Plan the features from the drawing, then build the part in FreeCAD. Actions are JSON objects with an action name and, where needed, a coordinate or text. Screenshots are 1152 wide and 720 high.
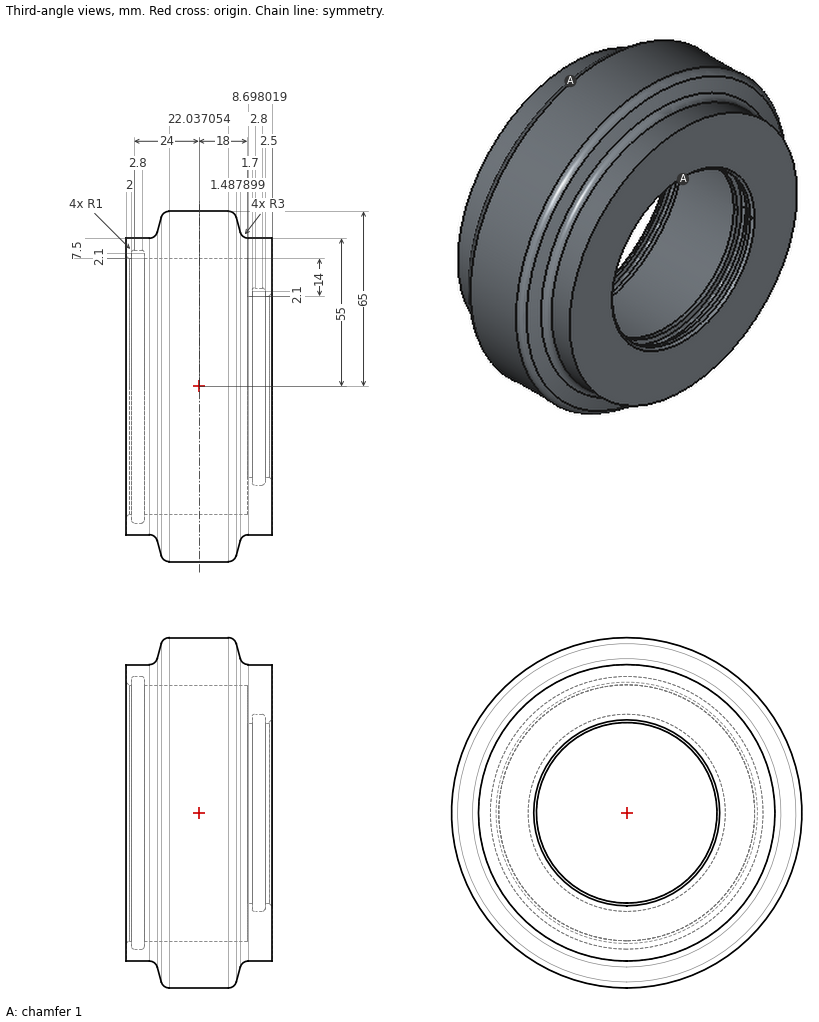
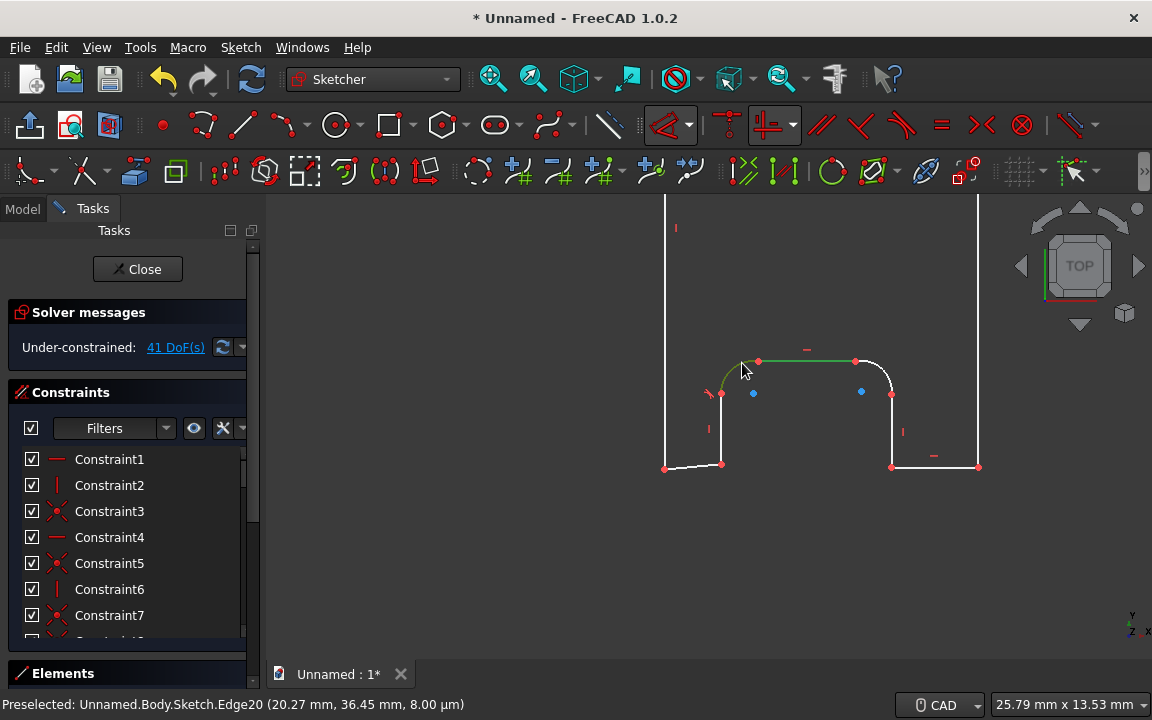
{"action": "key", "text": "t"}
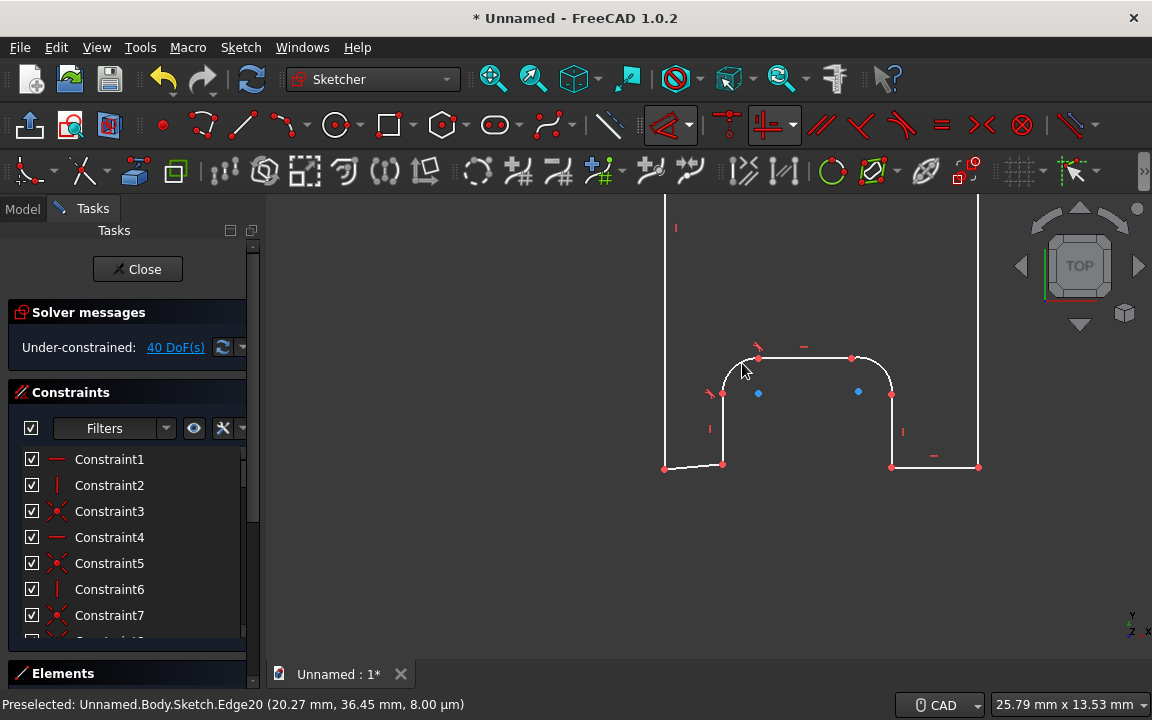
{"action": "left_click", "coordinate": [786, 358]}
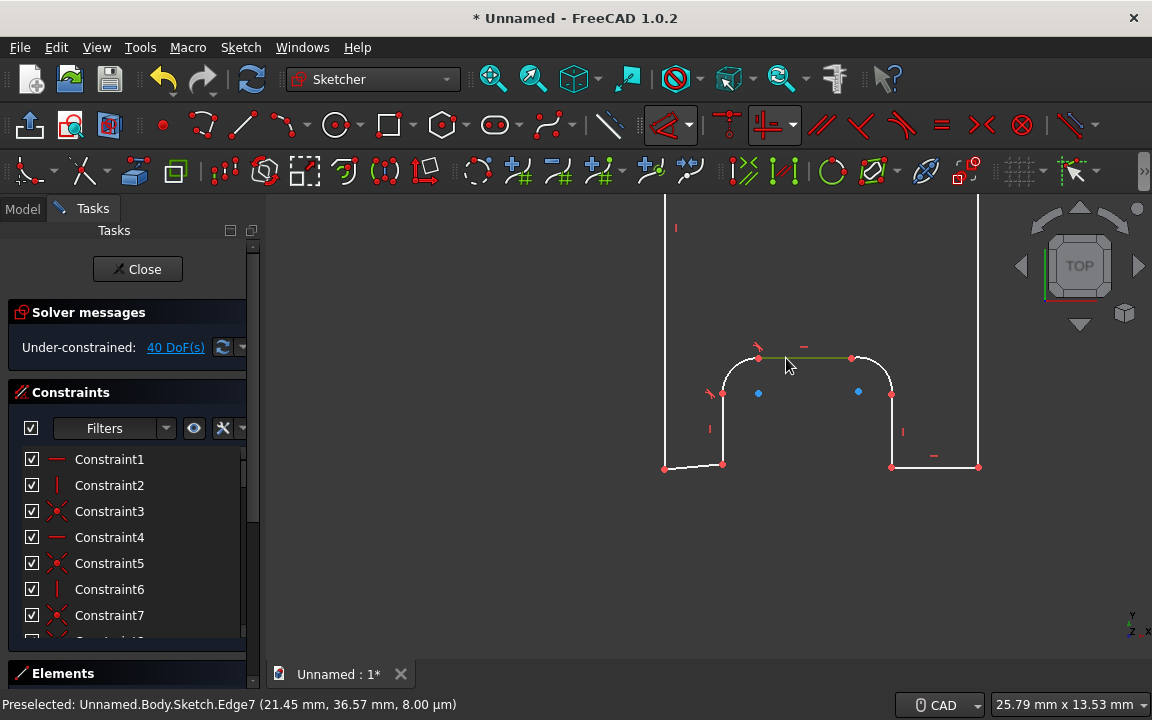
{"action": "left_click", "coordinate": [888, 376]}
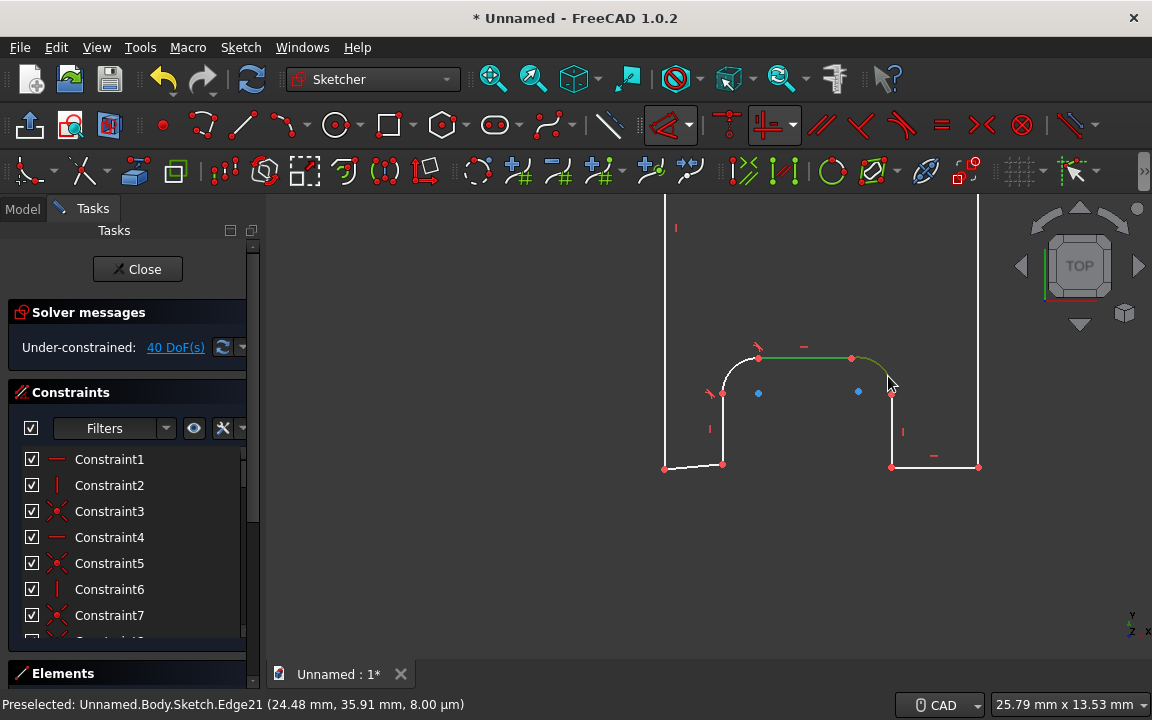
{"action": "key", "text": "t"}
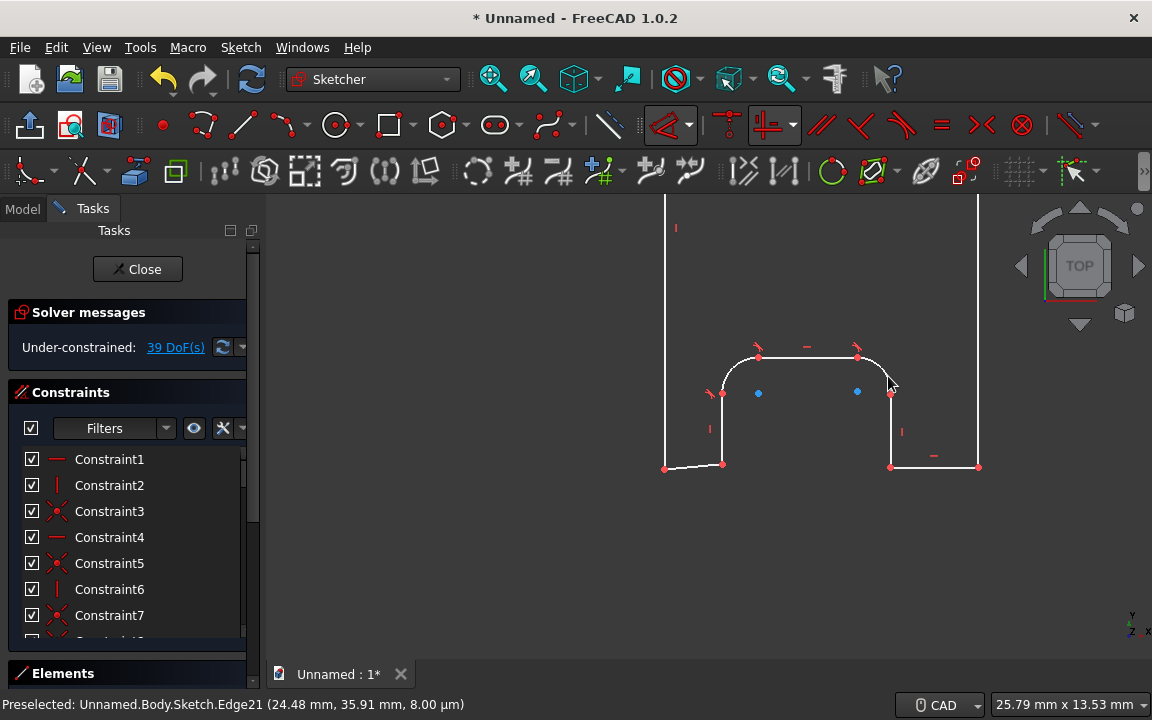
{"action": "left_click", "coordinate": [891, 417]}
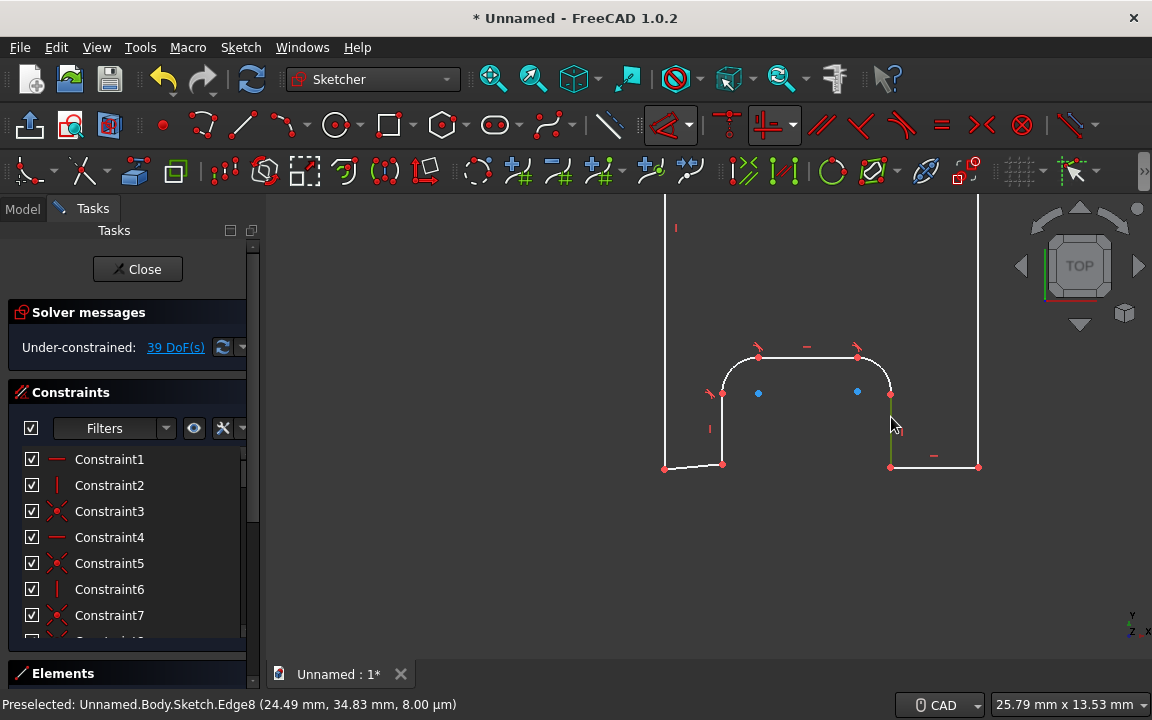
{"action": "left_click", "coordinate": [888, 378]}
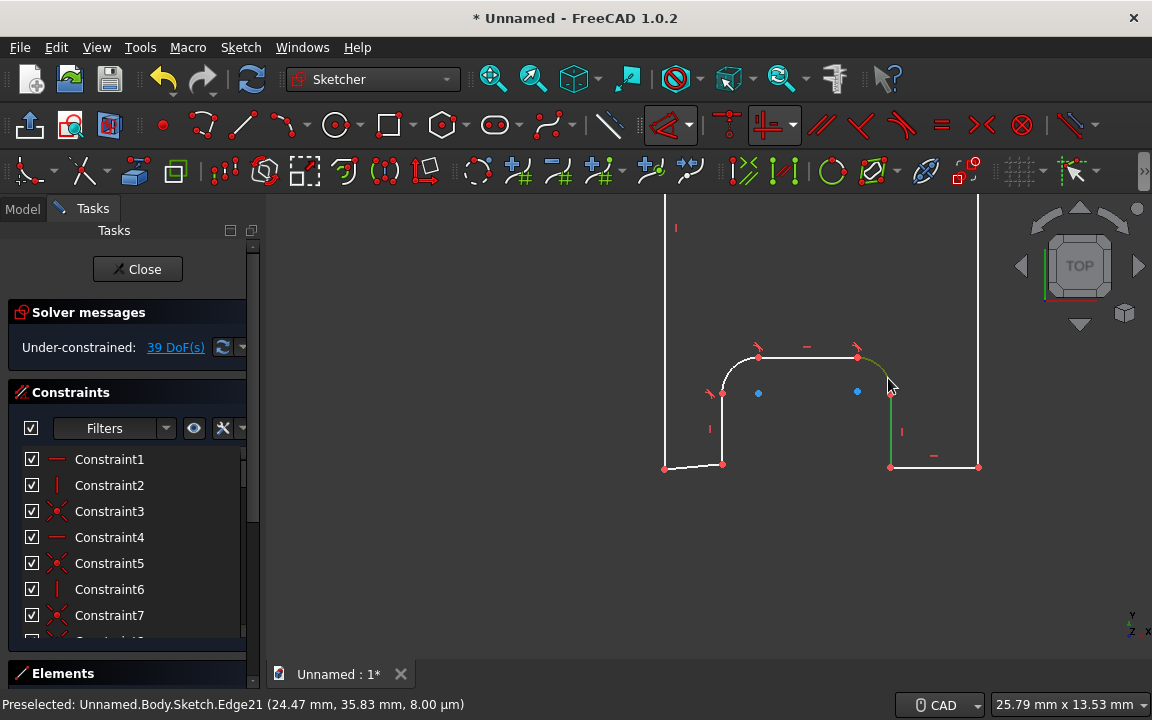
{"action": "key", "text": "t"}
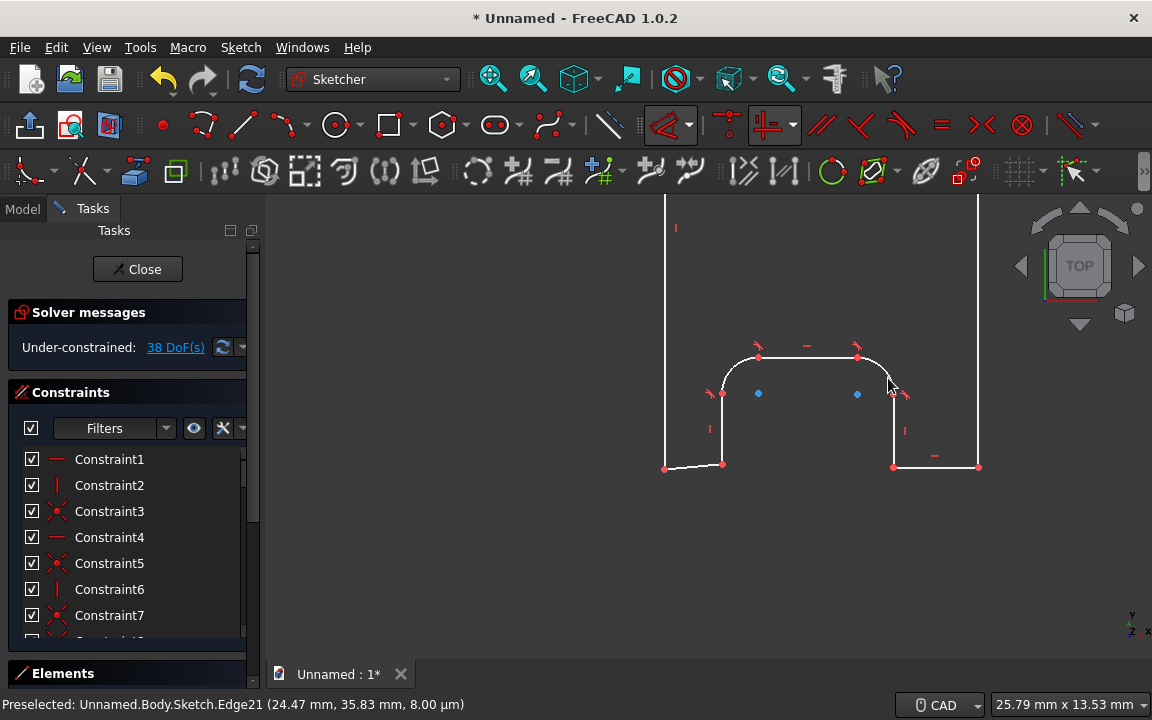
{"action": "scroll", "coordinate": [733, 415], "scroll_direction": "down", "scroll_amount": 10}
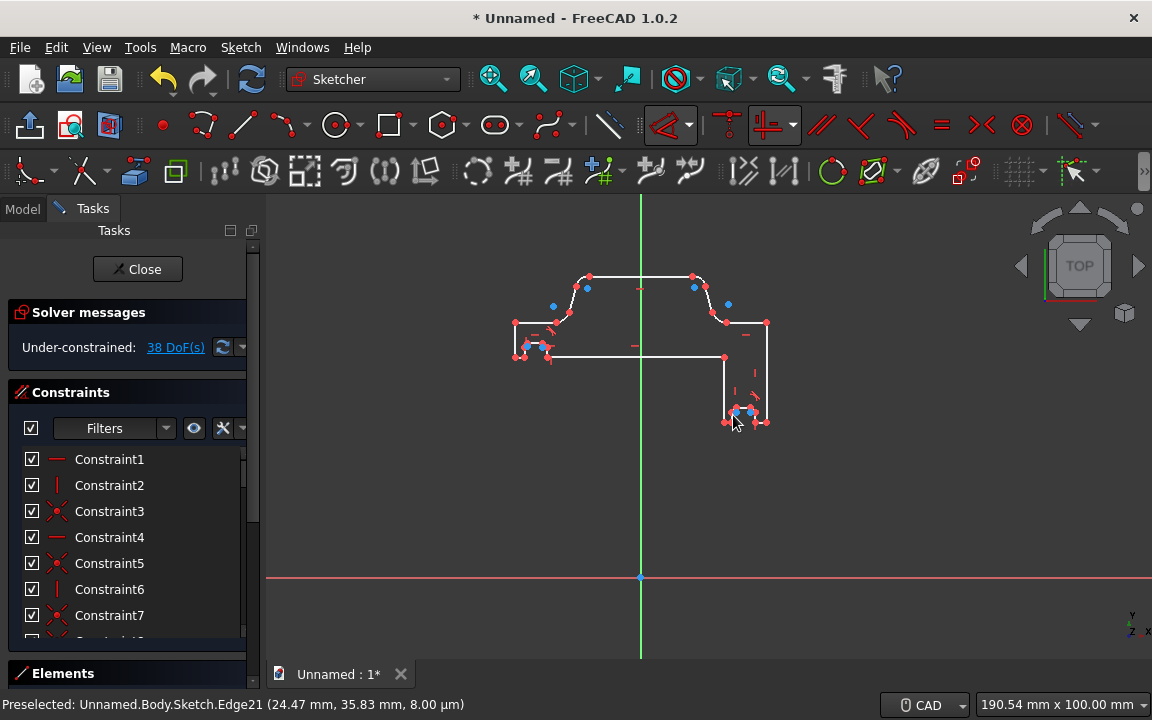
{"action": "left_click", "coordinate": [754, 323]}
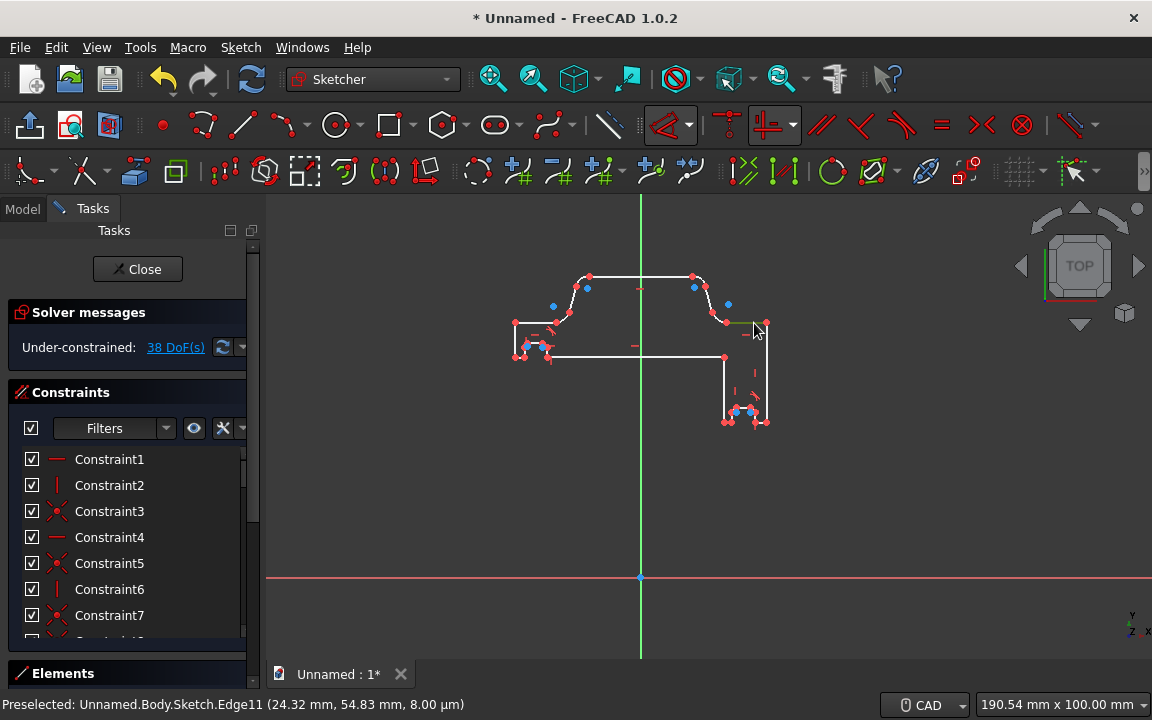
{"action": "scroll", "coordinate": [718, 320], "scroll_direction": "up", "scroll_amount": 3}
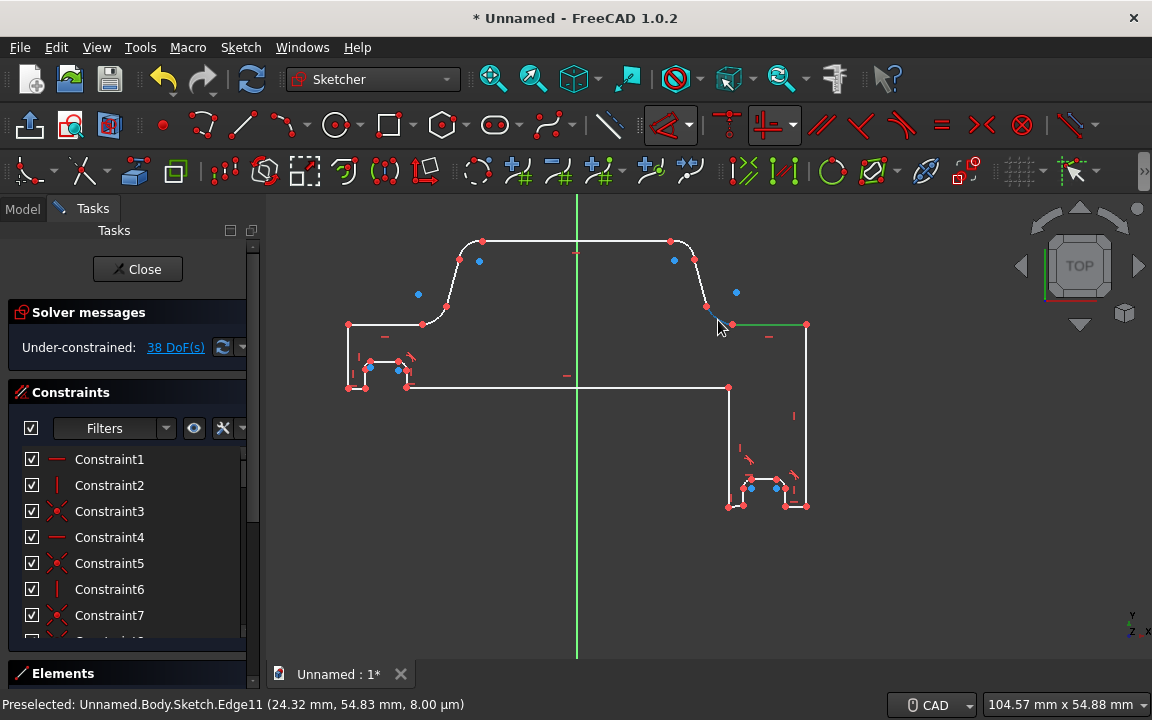
{"action": "left_click", "coordinate": [717, 319]}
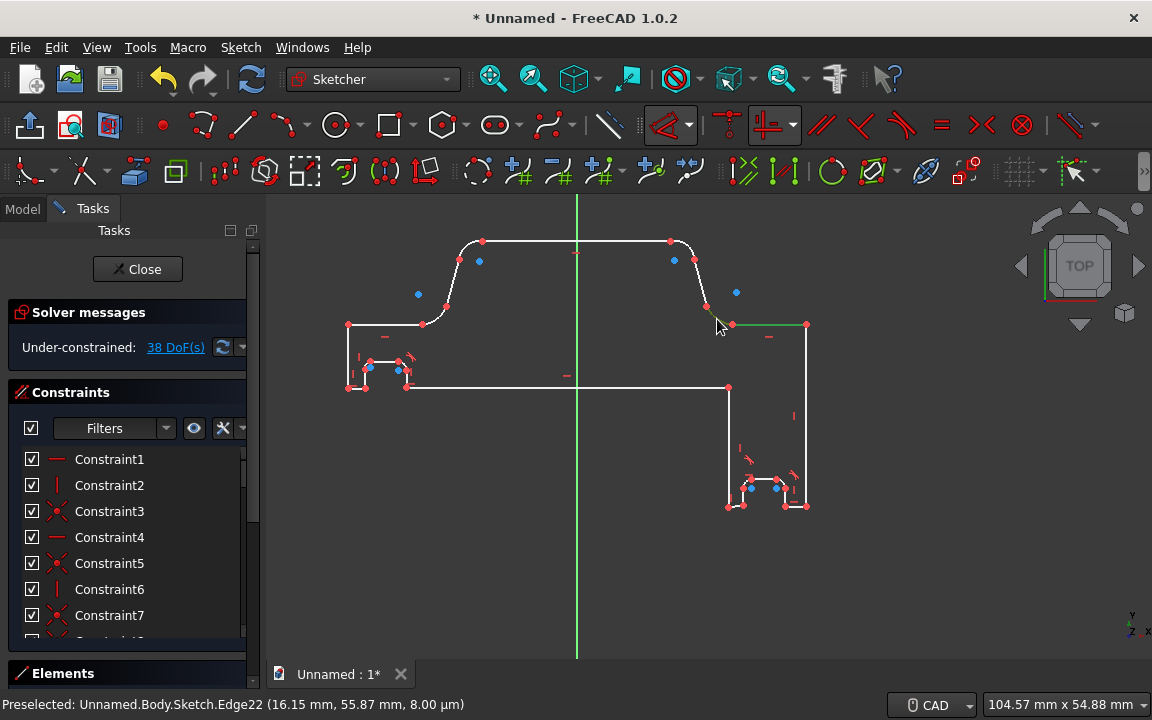
{"action": "left_click", "coordinate": [902, 126]}